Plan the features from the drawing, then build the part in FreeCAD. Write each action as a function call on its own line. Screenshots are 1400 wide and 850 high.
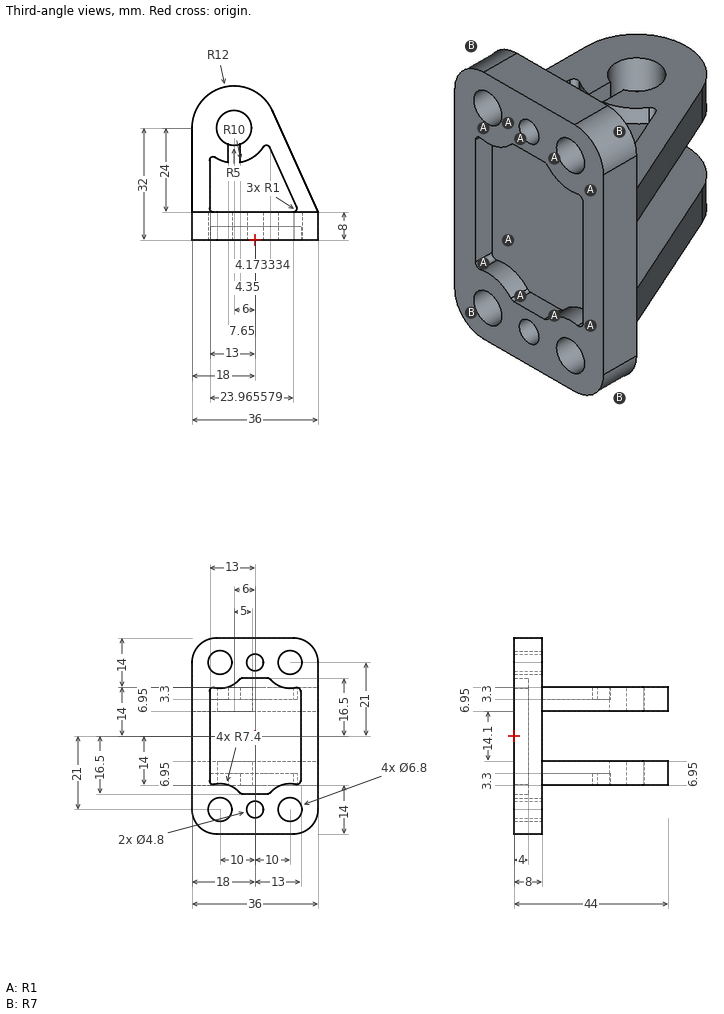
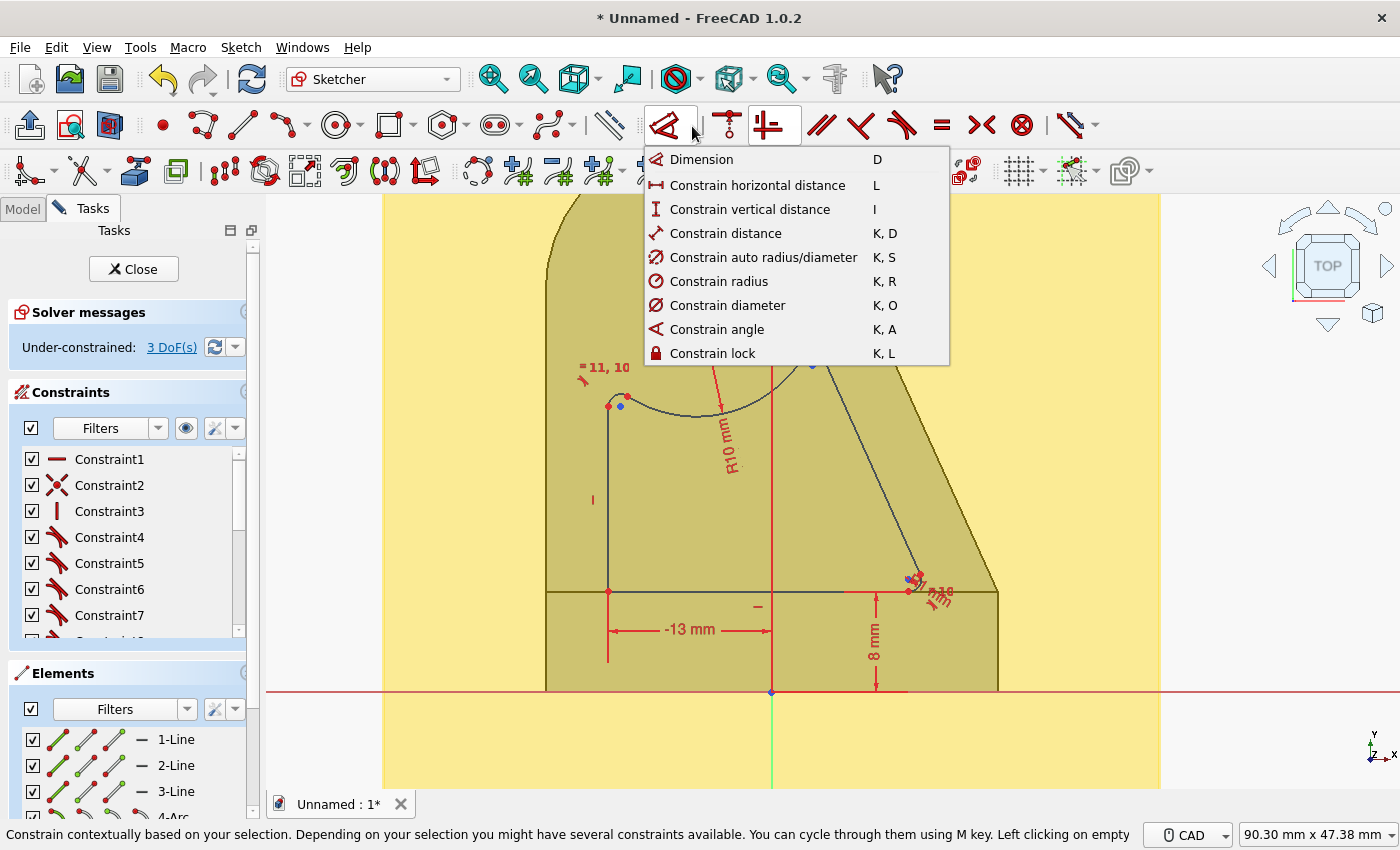
click(797, 209)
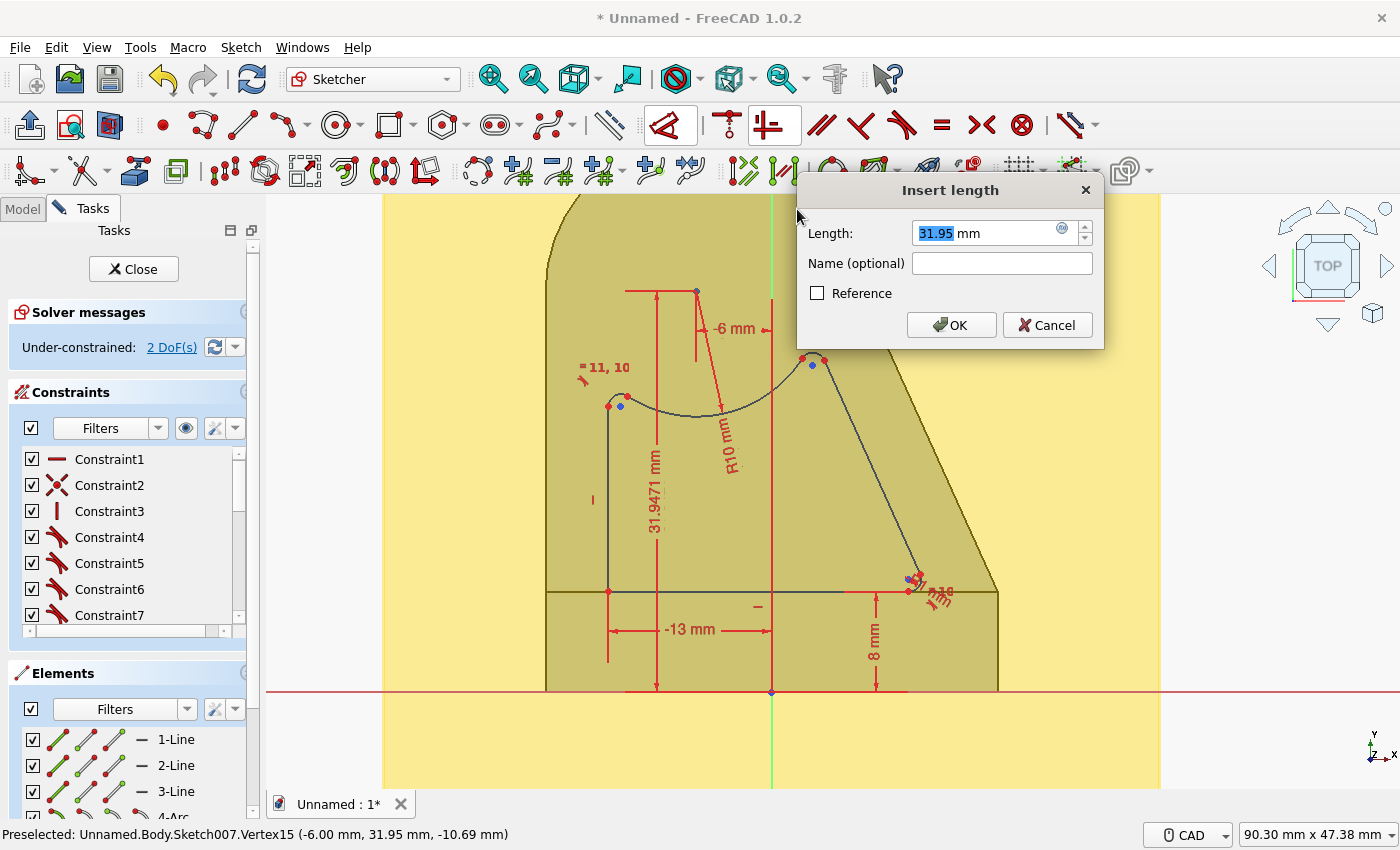
text(32)
key(Return)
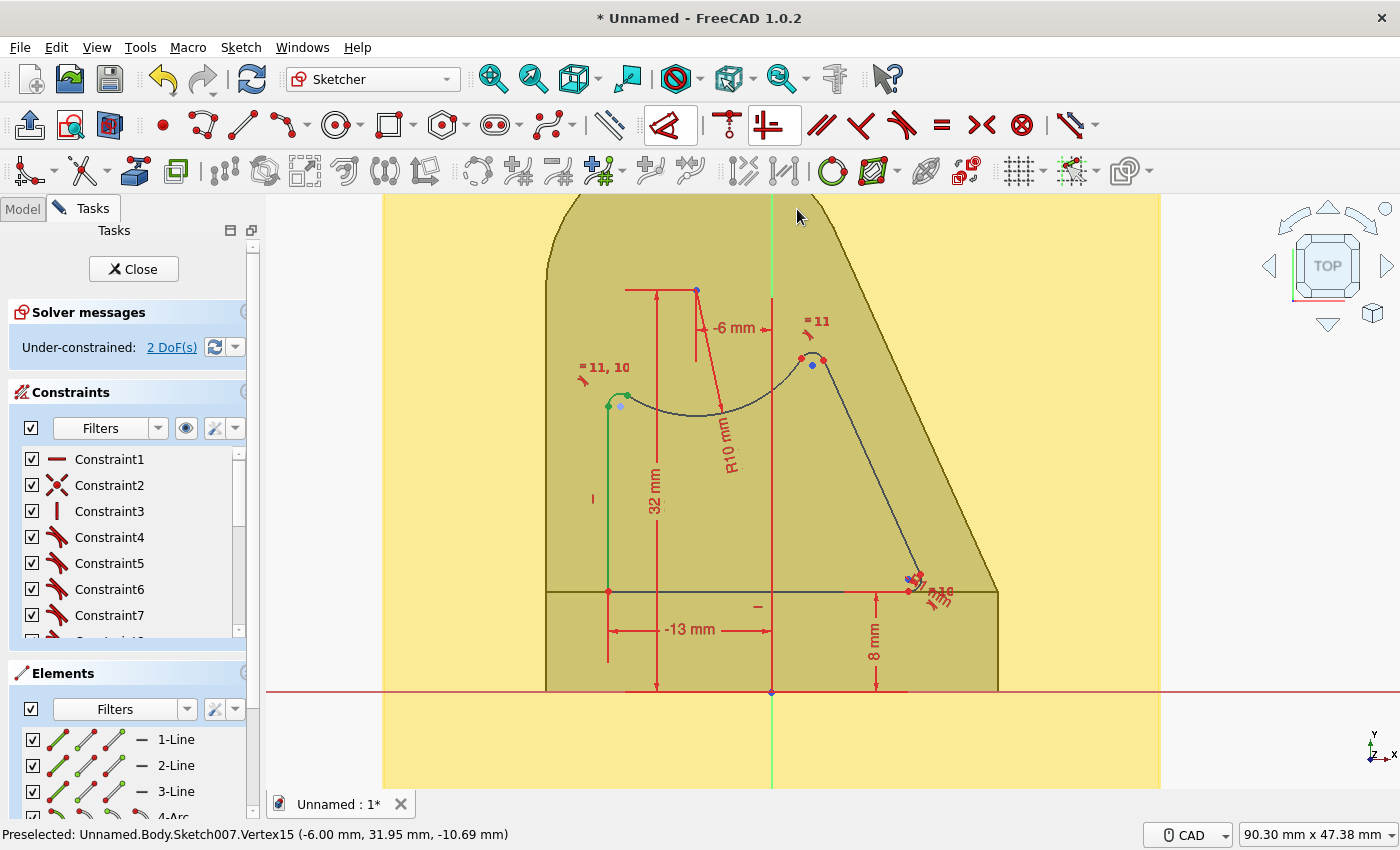
click(819, 592)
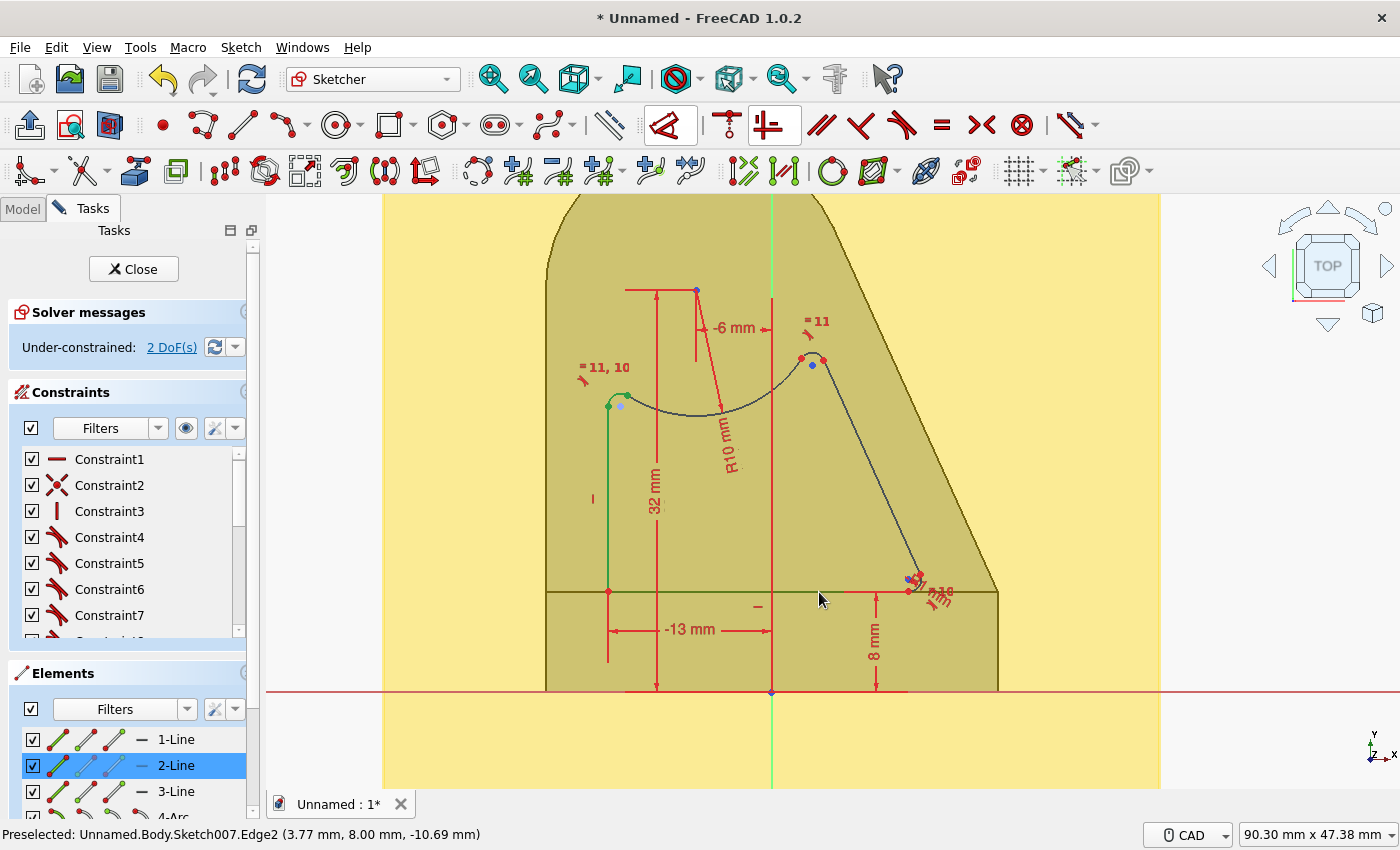
key(l)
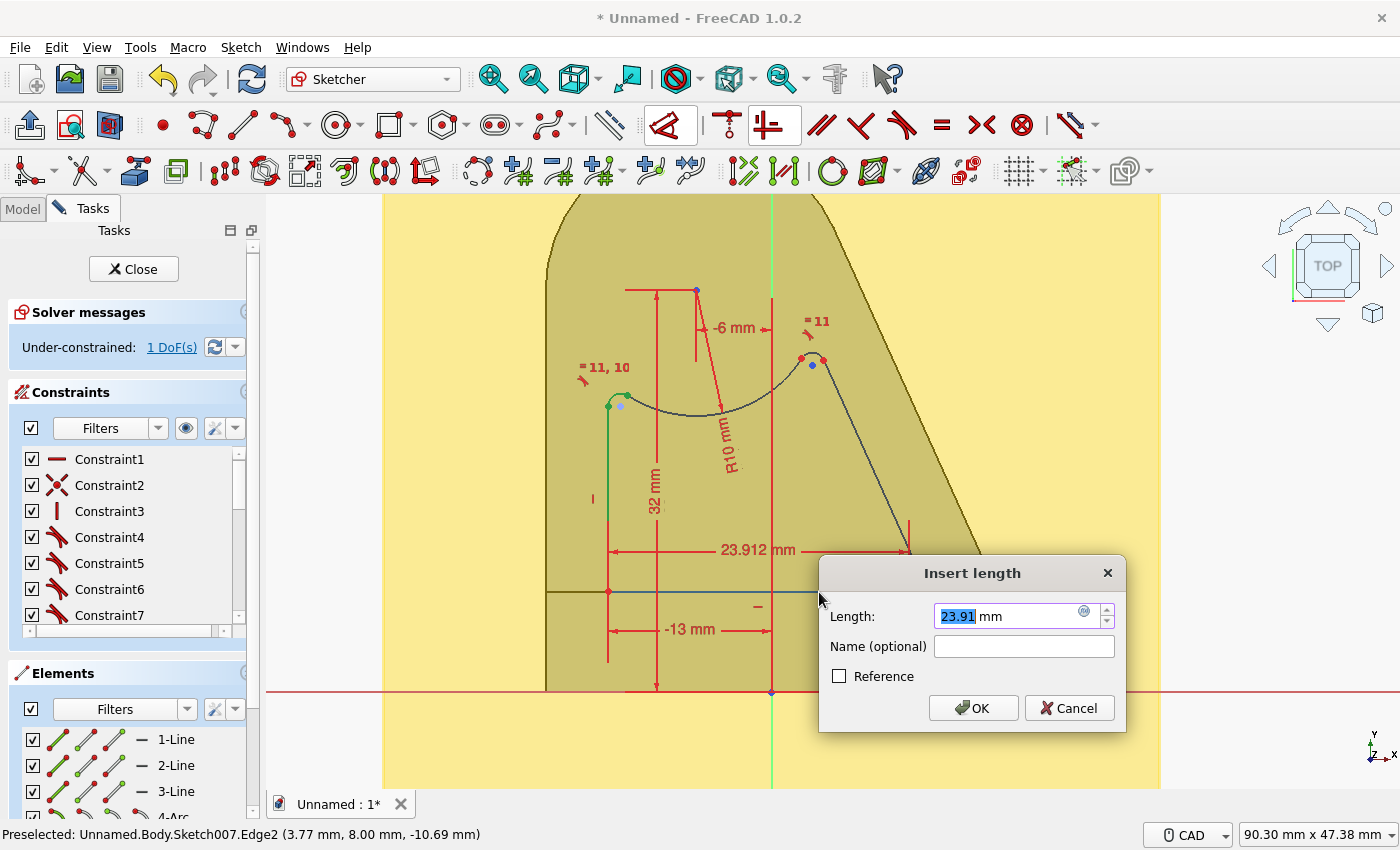
text(23.965579)
key(Return)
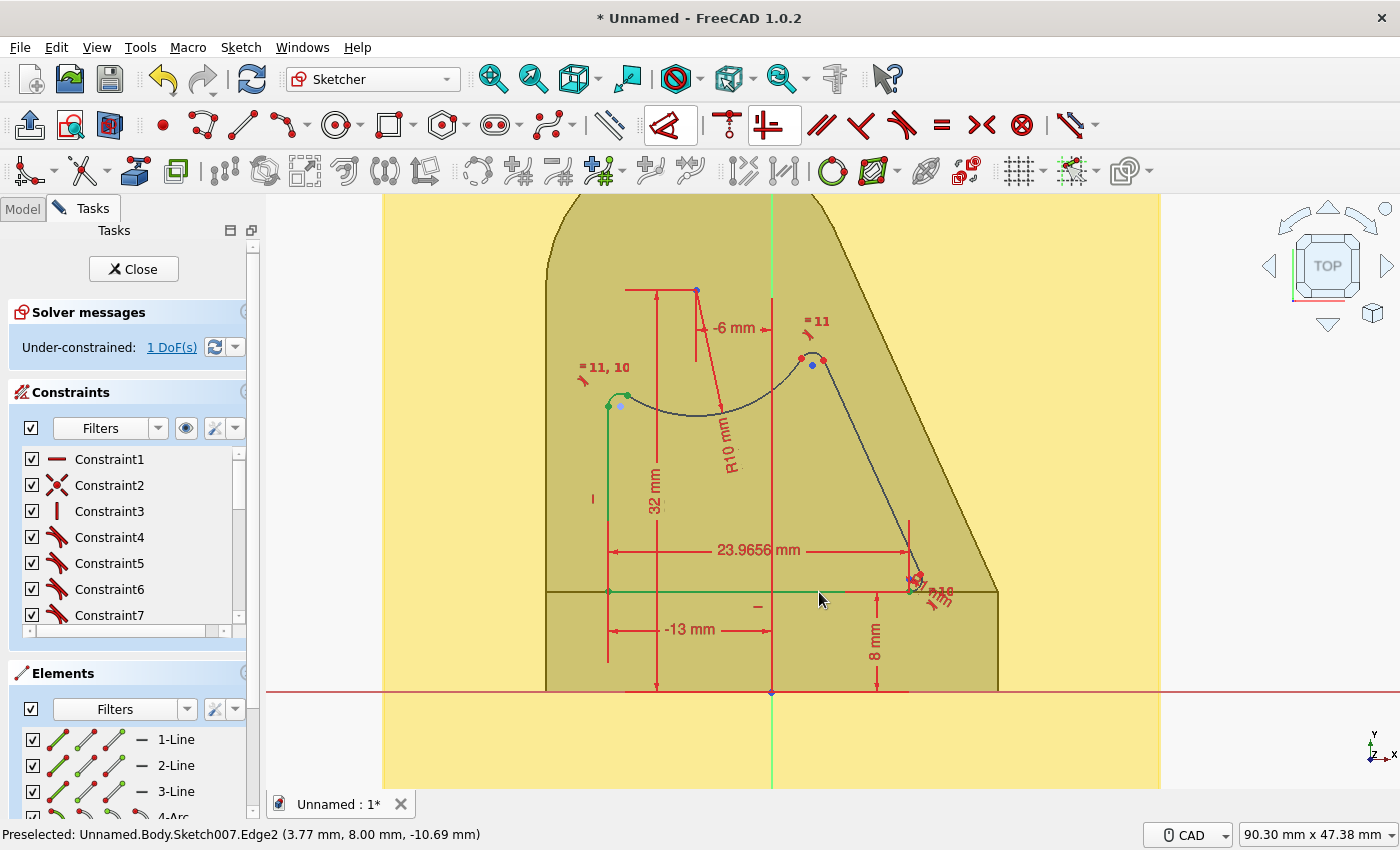
click(824, 360)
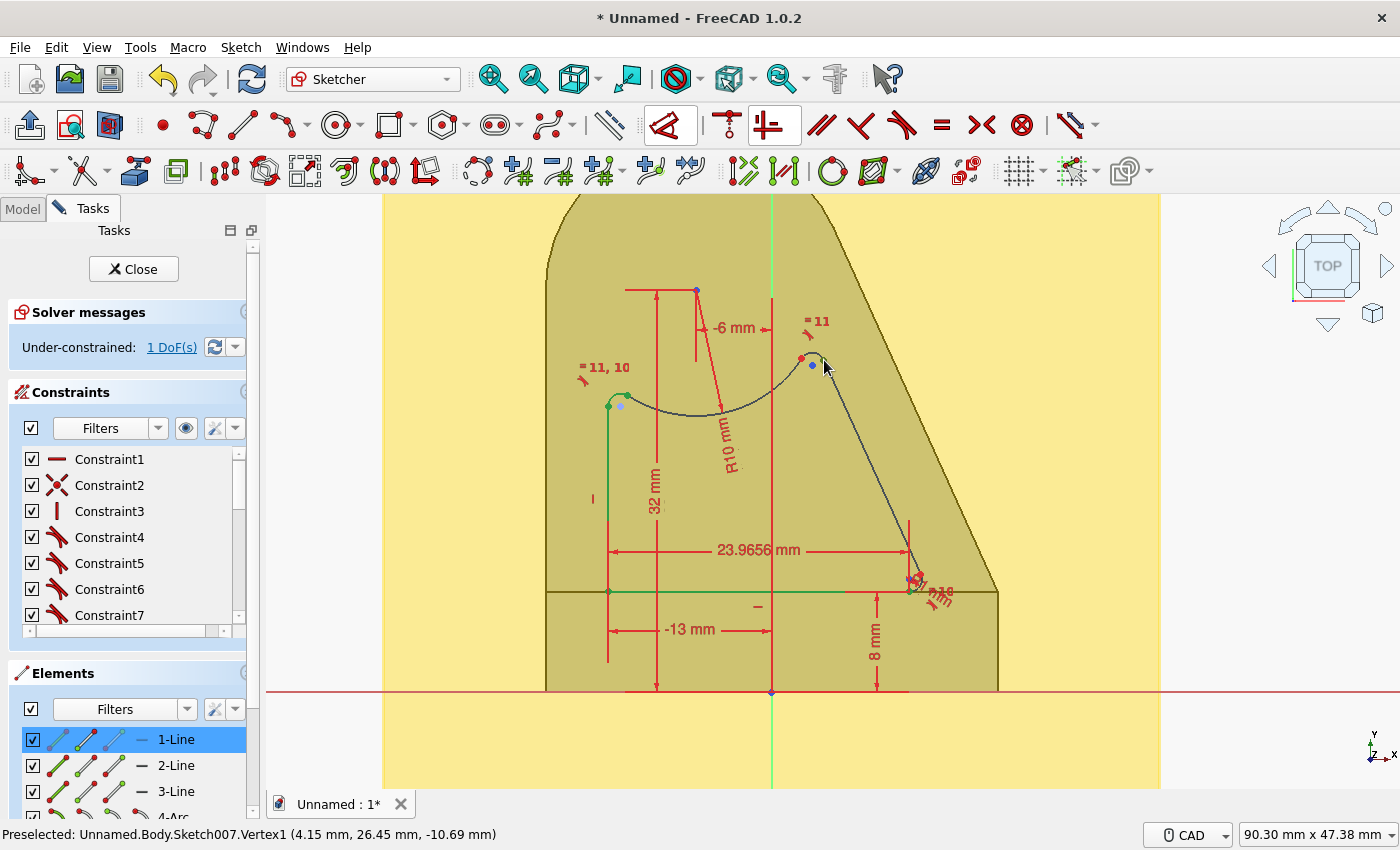
click(692, 126)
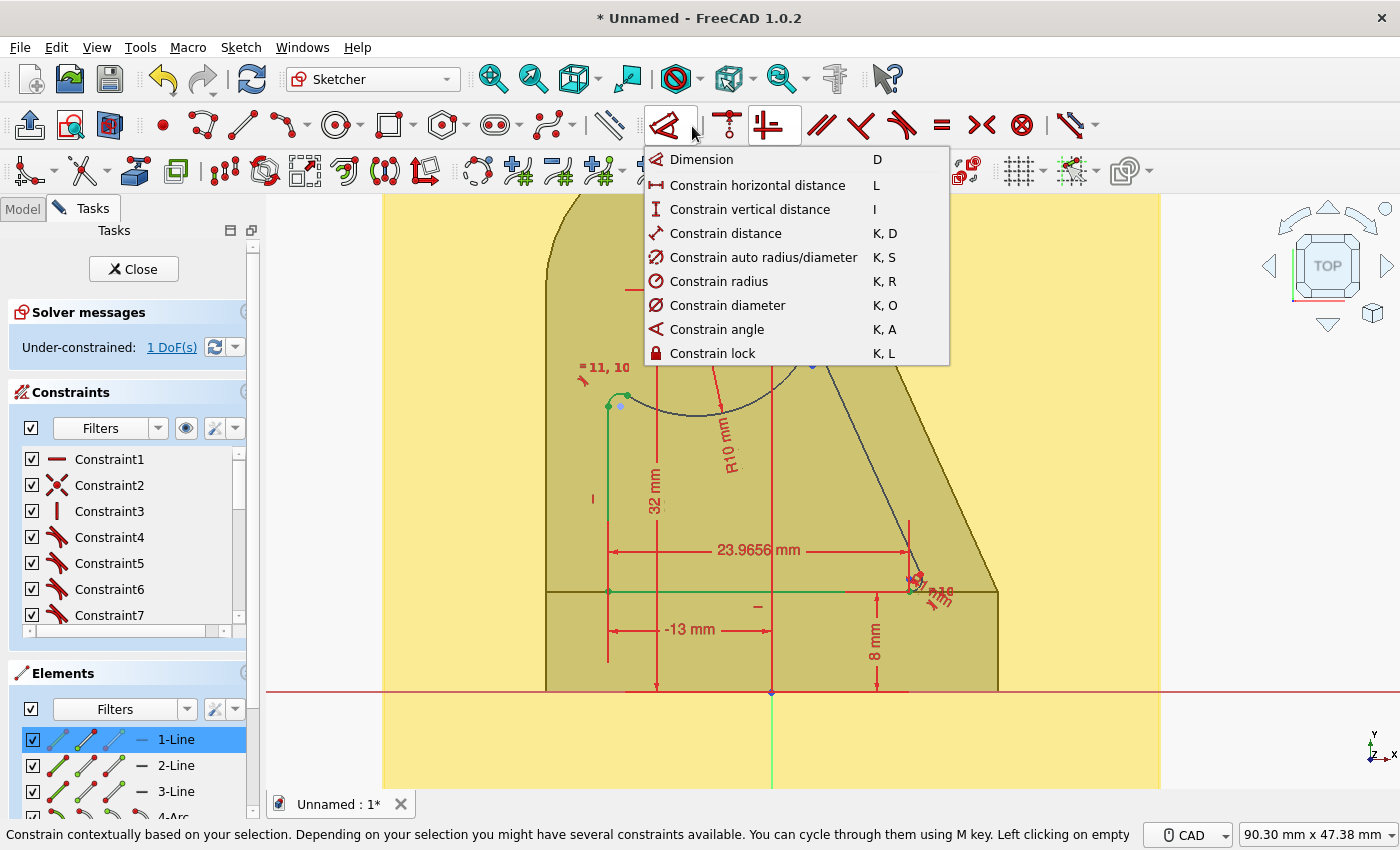
click(797, 185)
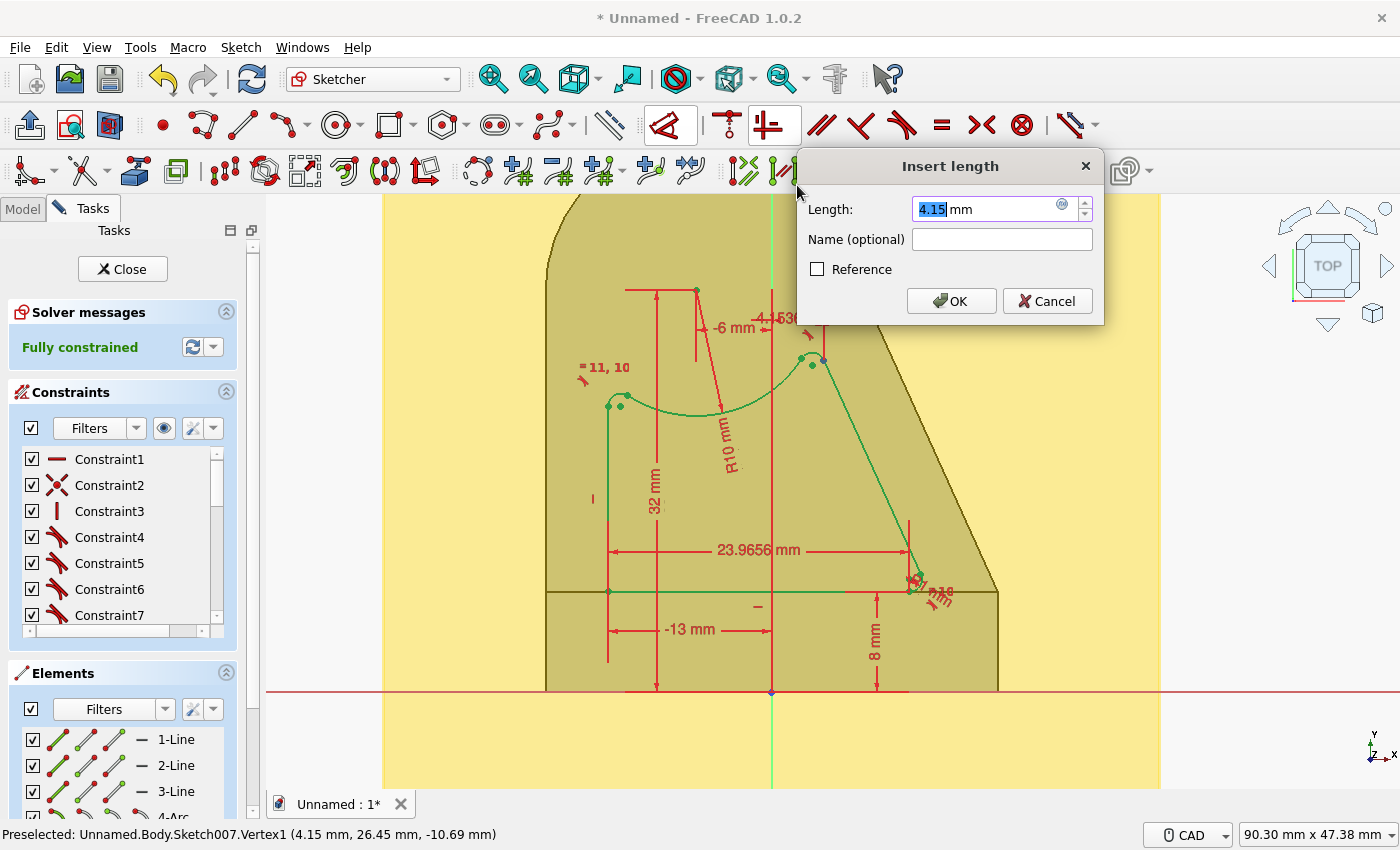
text(4.173334)
key(Return)